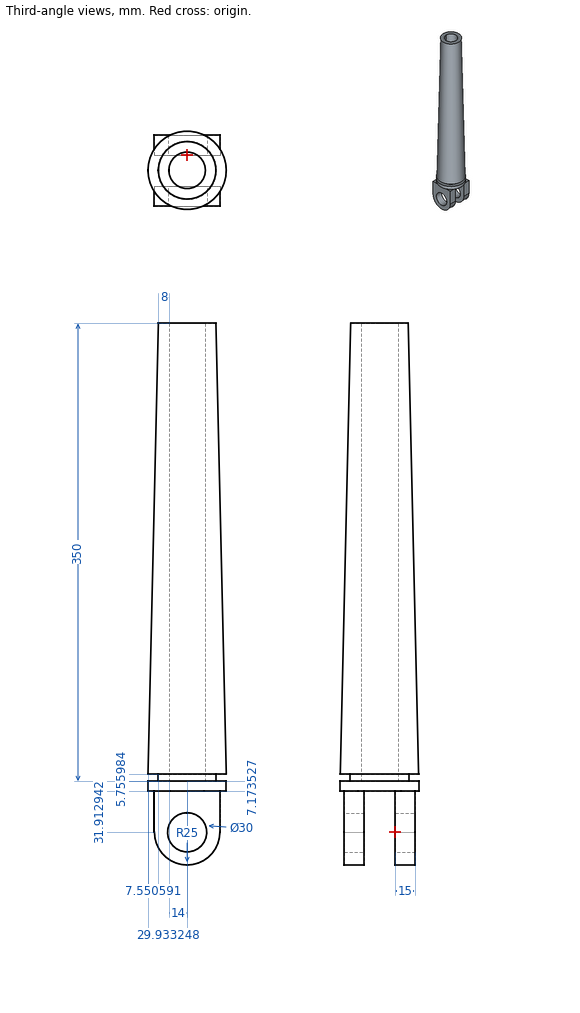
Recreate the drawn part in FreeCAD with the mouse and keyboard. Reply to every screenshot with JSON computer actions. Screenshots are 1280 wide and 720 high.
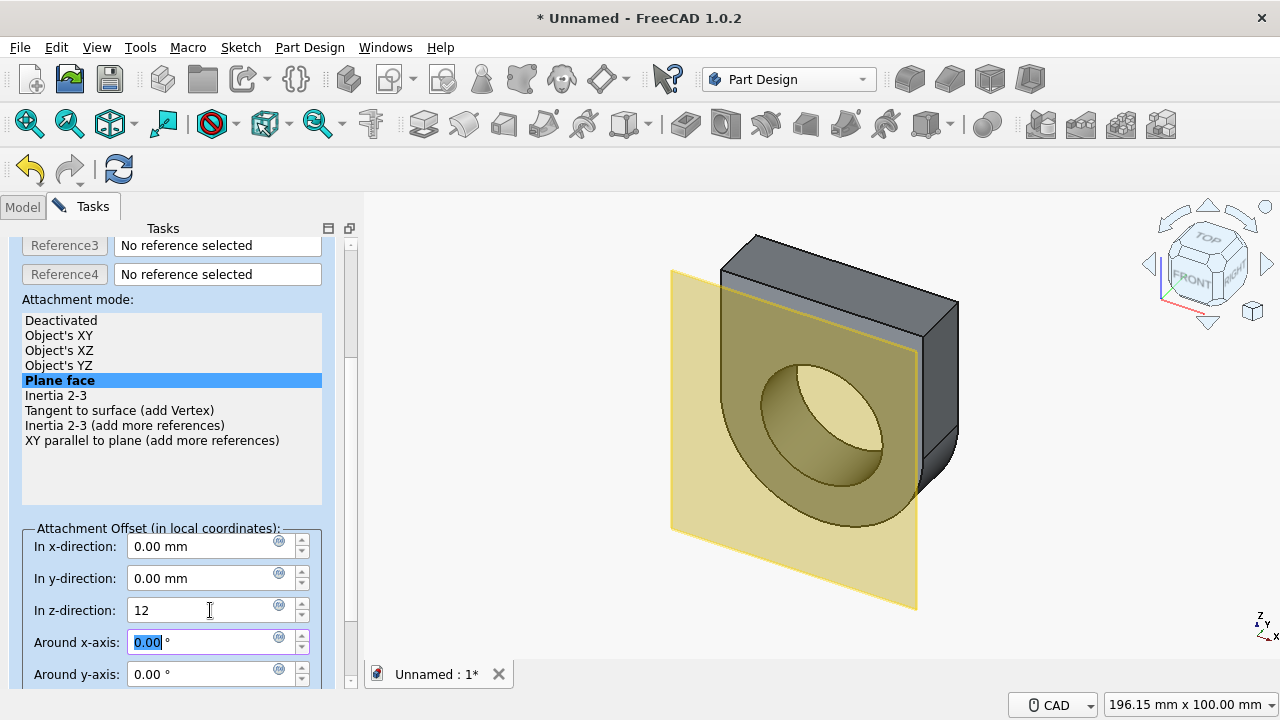
{"action": "scroll", "coordinate": [351, 463], "scroll_direction": "up", "scroll_amount": 4}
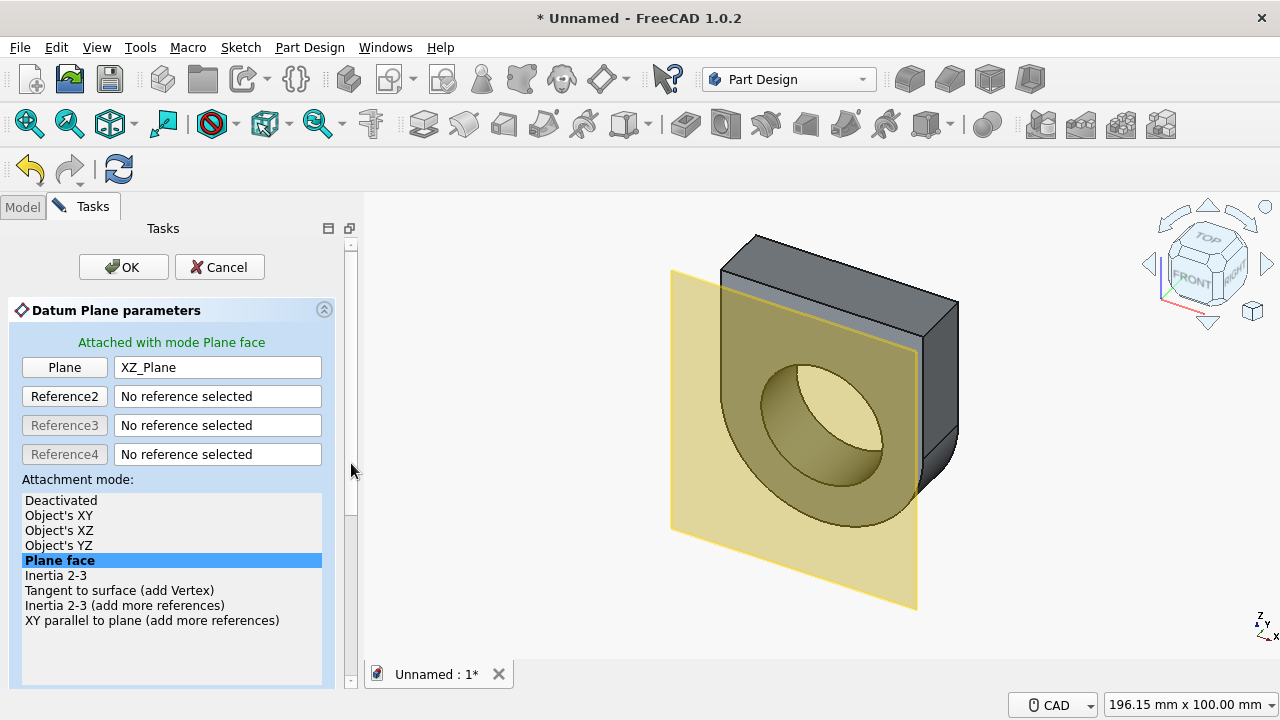
{"action": "left_click", "coordinate": [124, 267]}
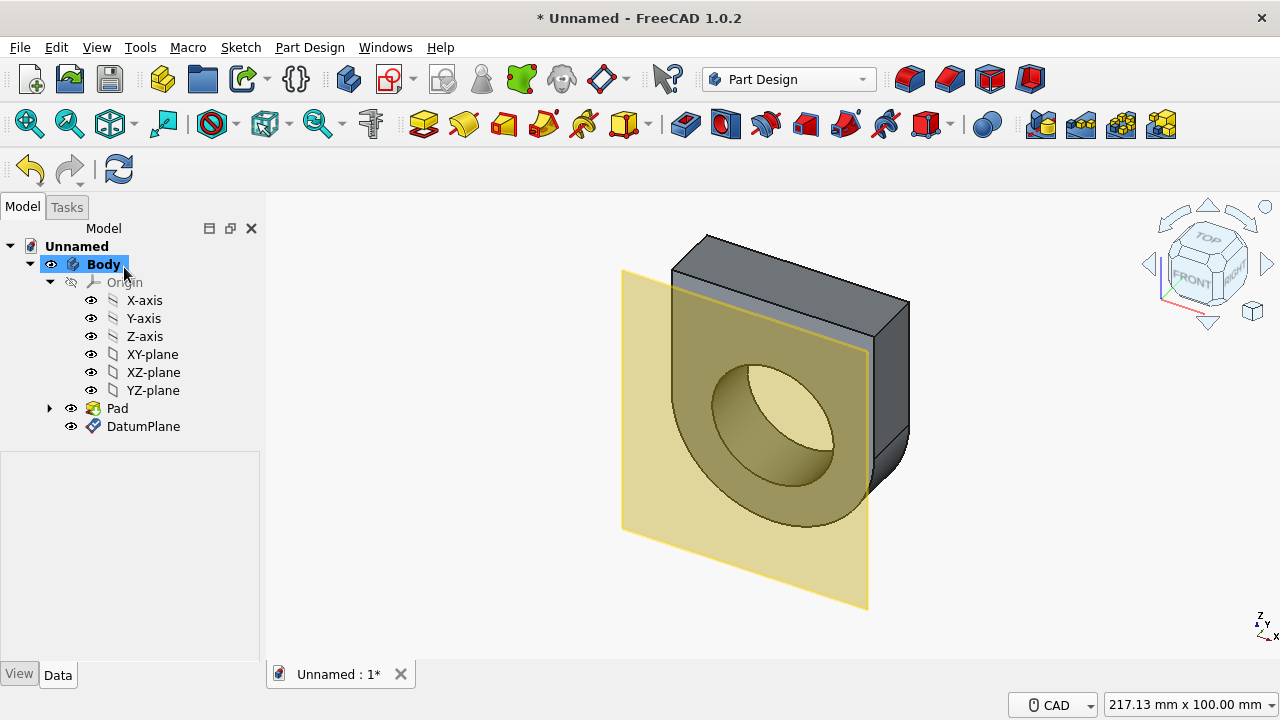
{"action": "left_click", "coordinate": [116, 426]}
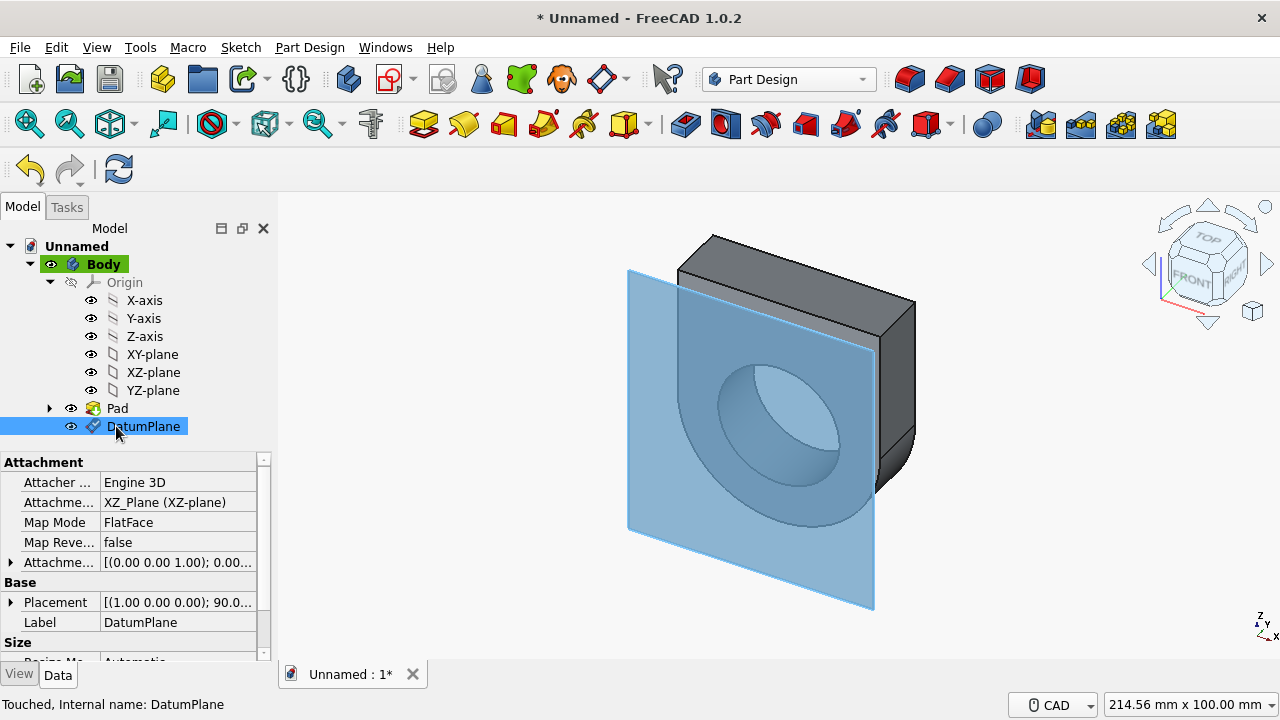
{"action": "left_click", "coordinate": [390, 80]}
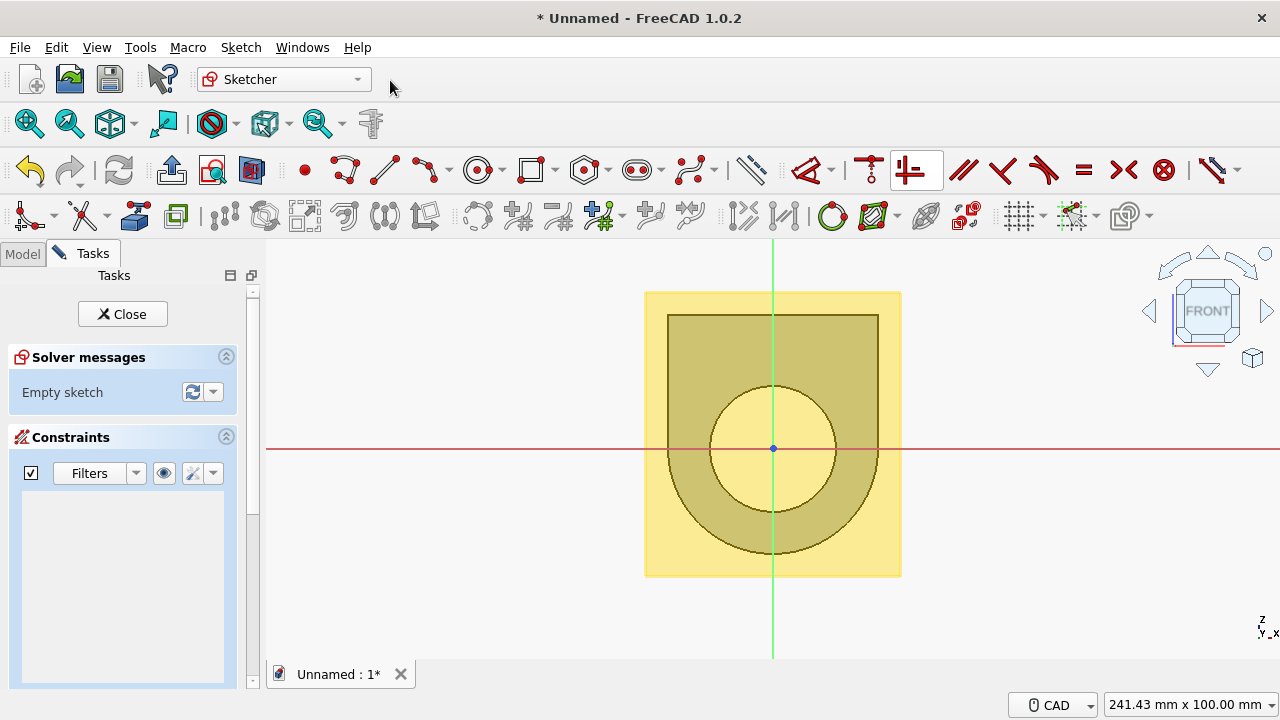
{"action": "scroll", "coordinate": [703, 611], "scroll_direction": "down", "scroll_amount": 9}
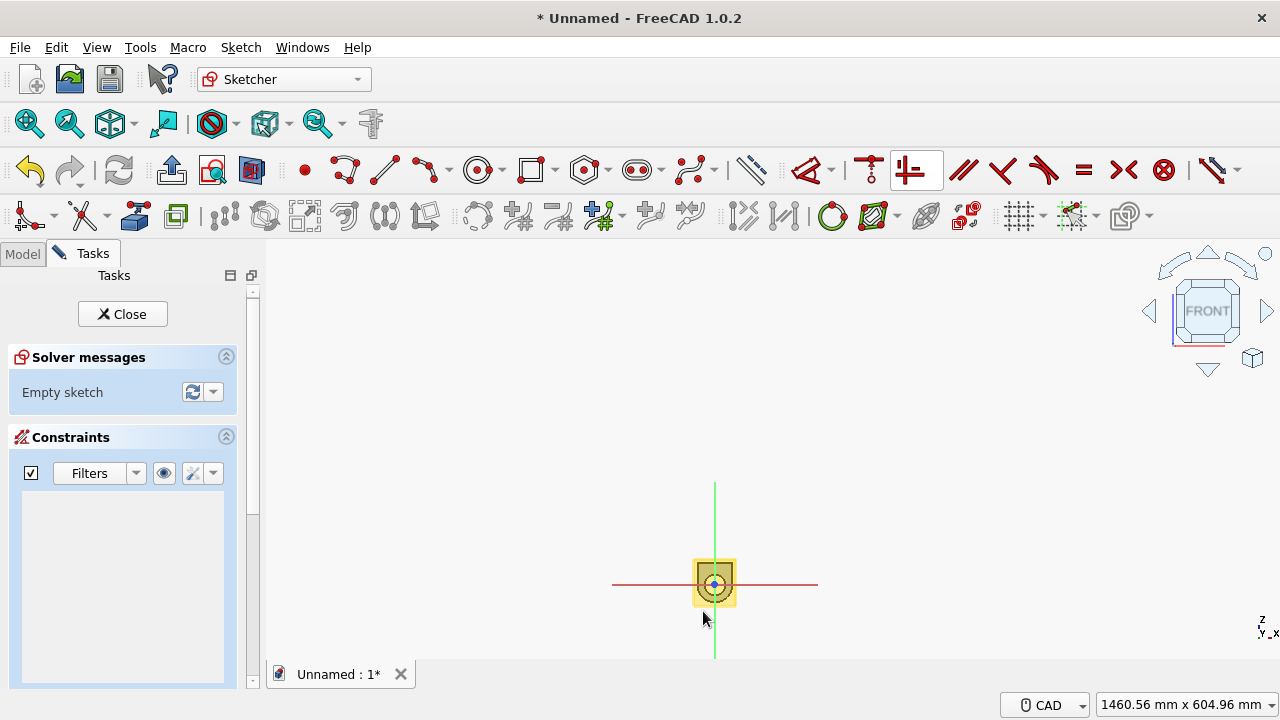
{"action": "left_click", "coordinate": [346, 170]}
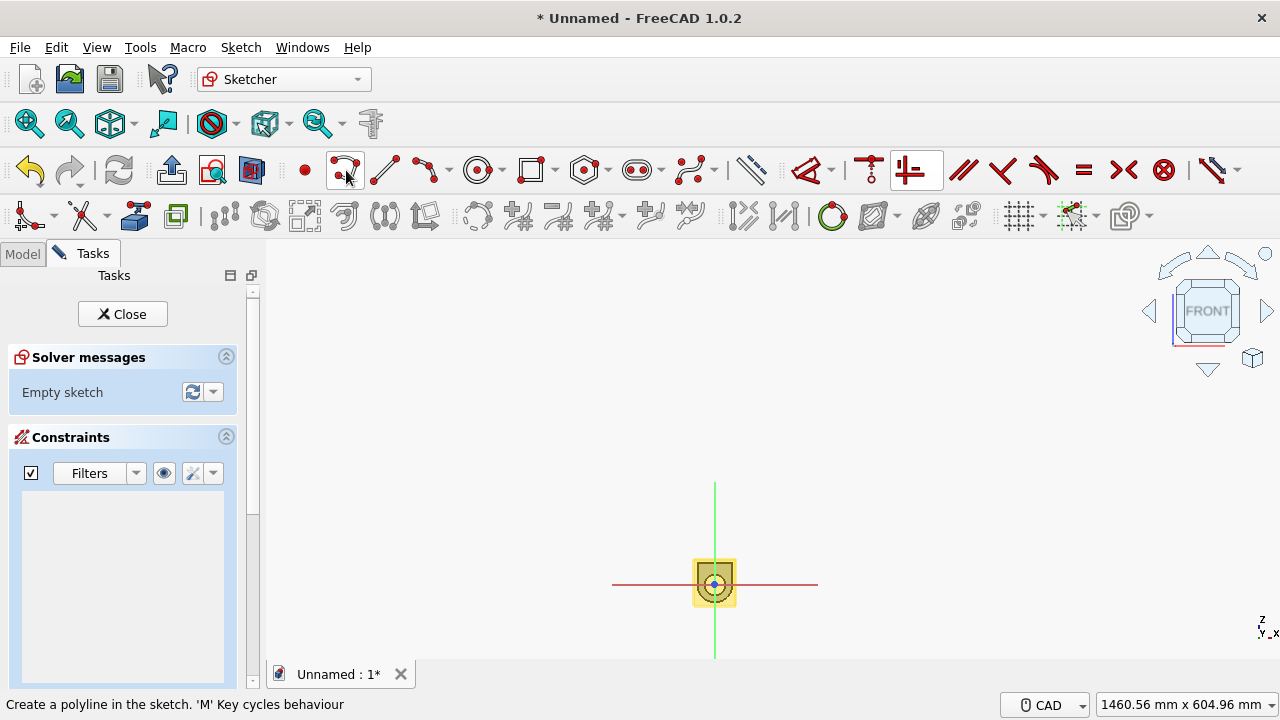
{"action": "left_click", "coordinate": [715, 563]}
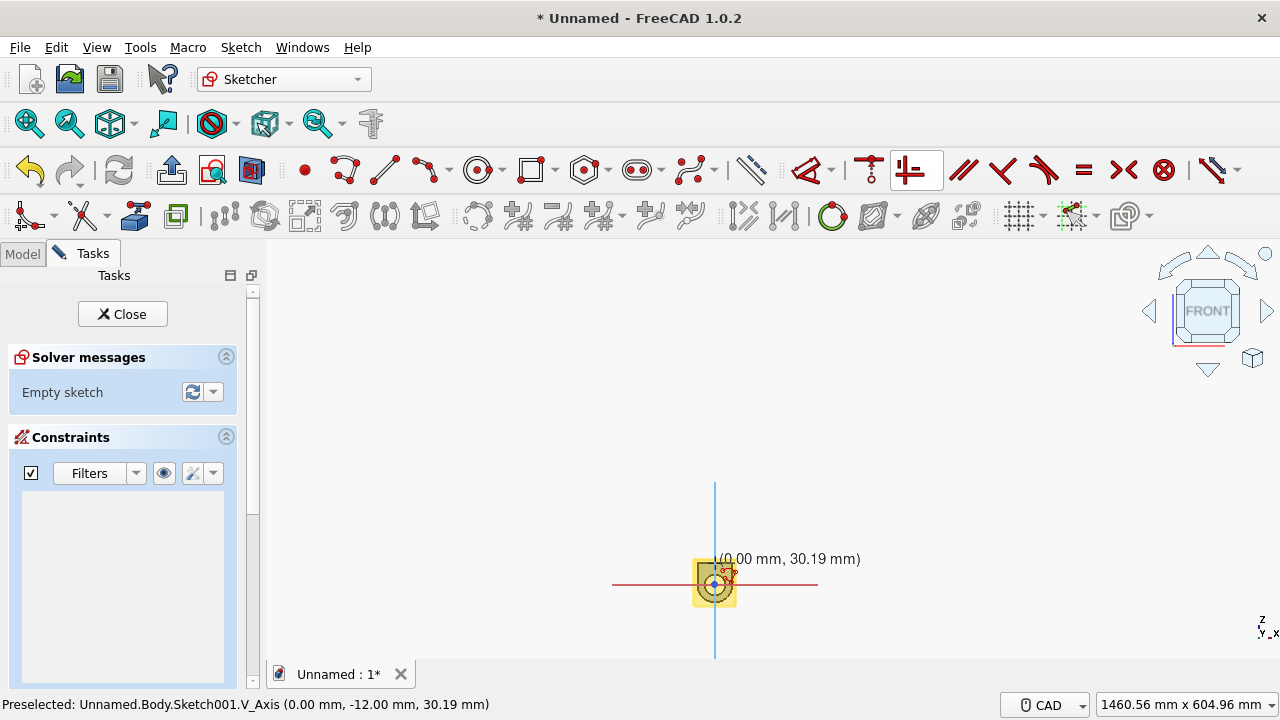
{"action": "scroll", "coordinate": [715, 558], "scroll_direction": "up", "scroll_amount": 6}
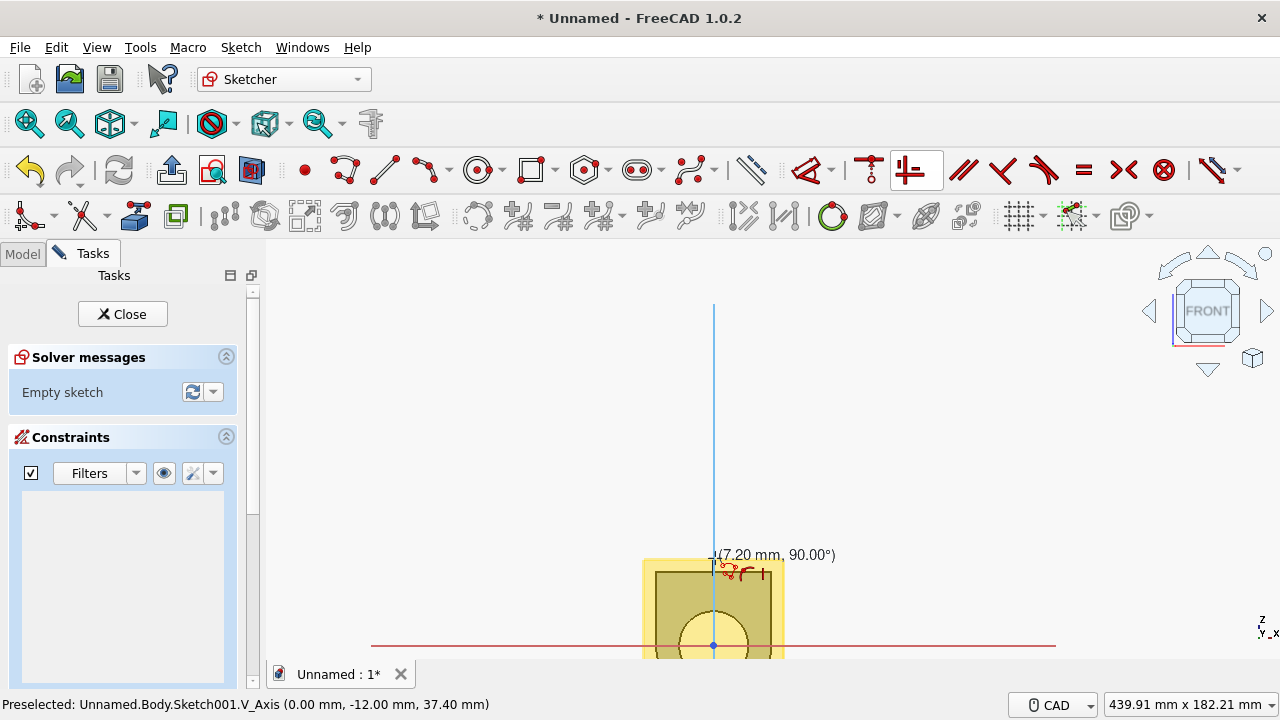
{"action": "left_click", "coordinate": [705, 556]}
{"action": "left_click", "coordinate": [681, 556]}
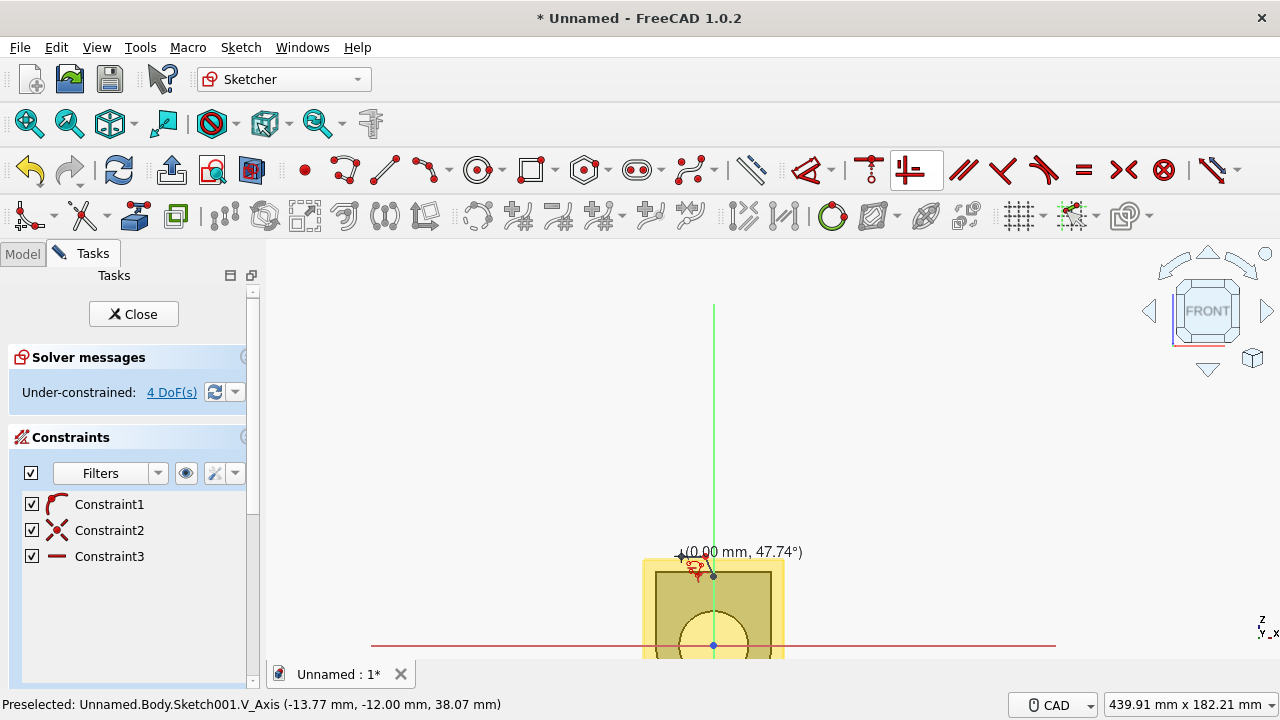
{"action": "scroll", "coordinate": [715, 557], "scroll_direction": "down", "scroll_amount": 6}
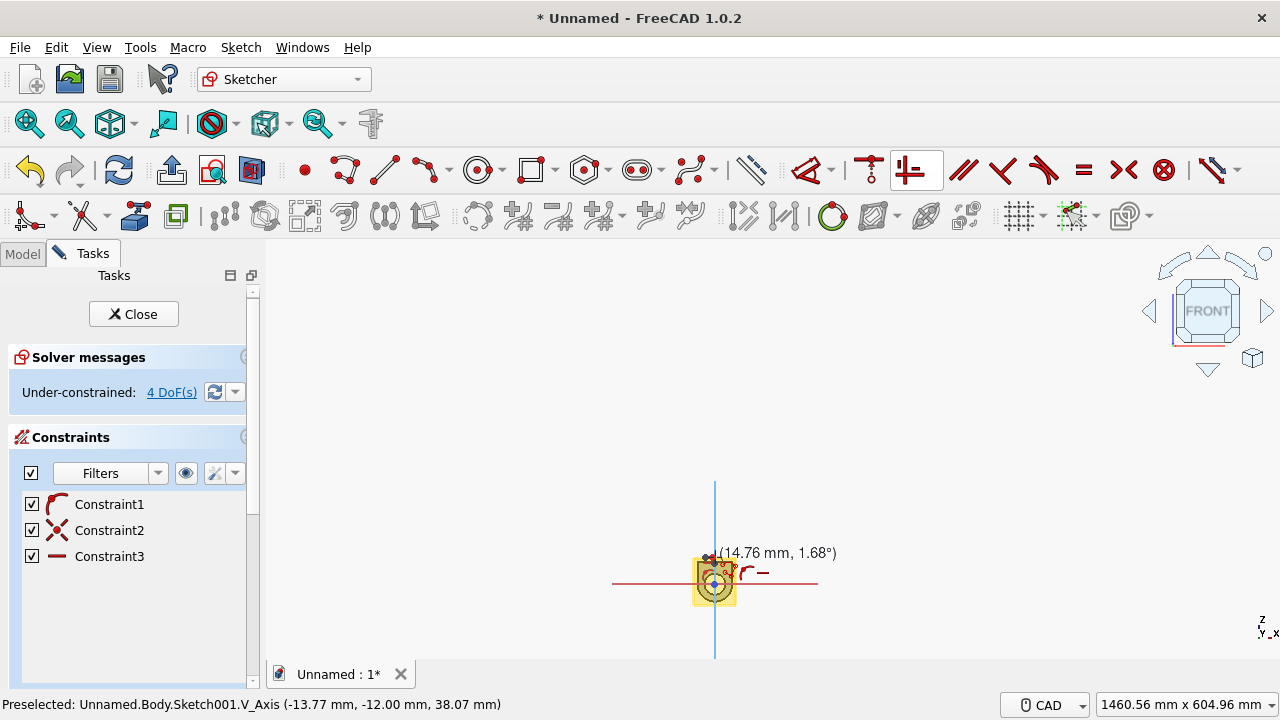
{"action": "scroll", "coordinate": [705, 314], "scroll_direction": "up", "scroll_amount": 3}